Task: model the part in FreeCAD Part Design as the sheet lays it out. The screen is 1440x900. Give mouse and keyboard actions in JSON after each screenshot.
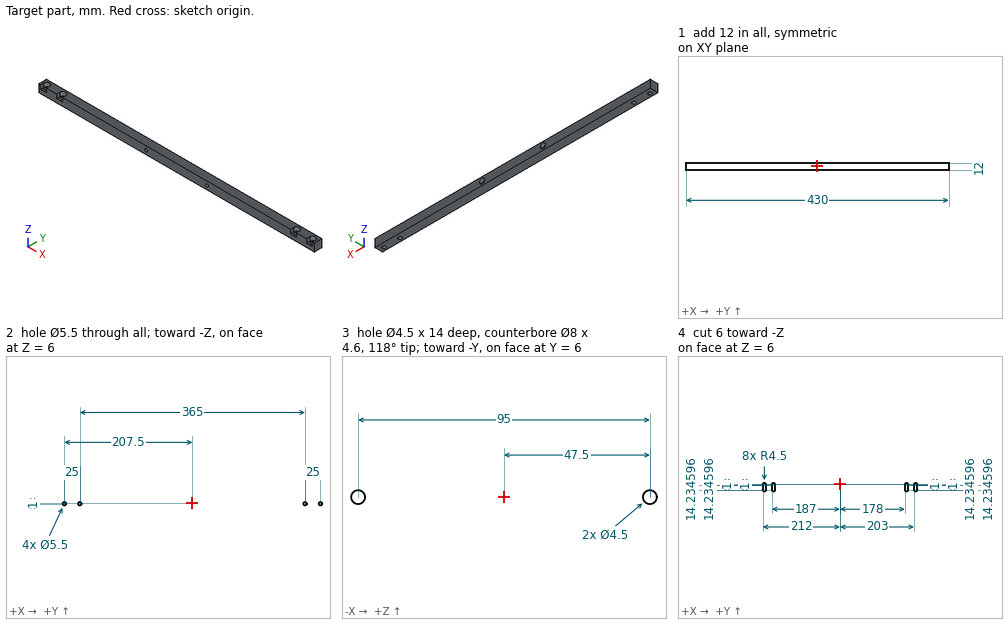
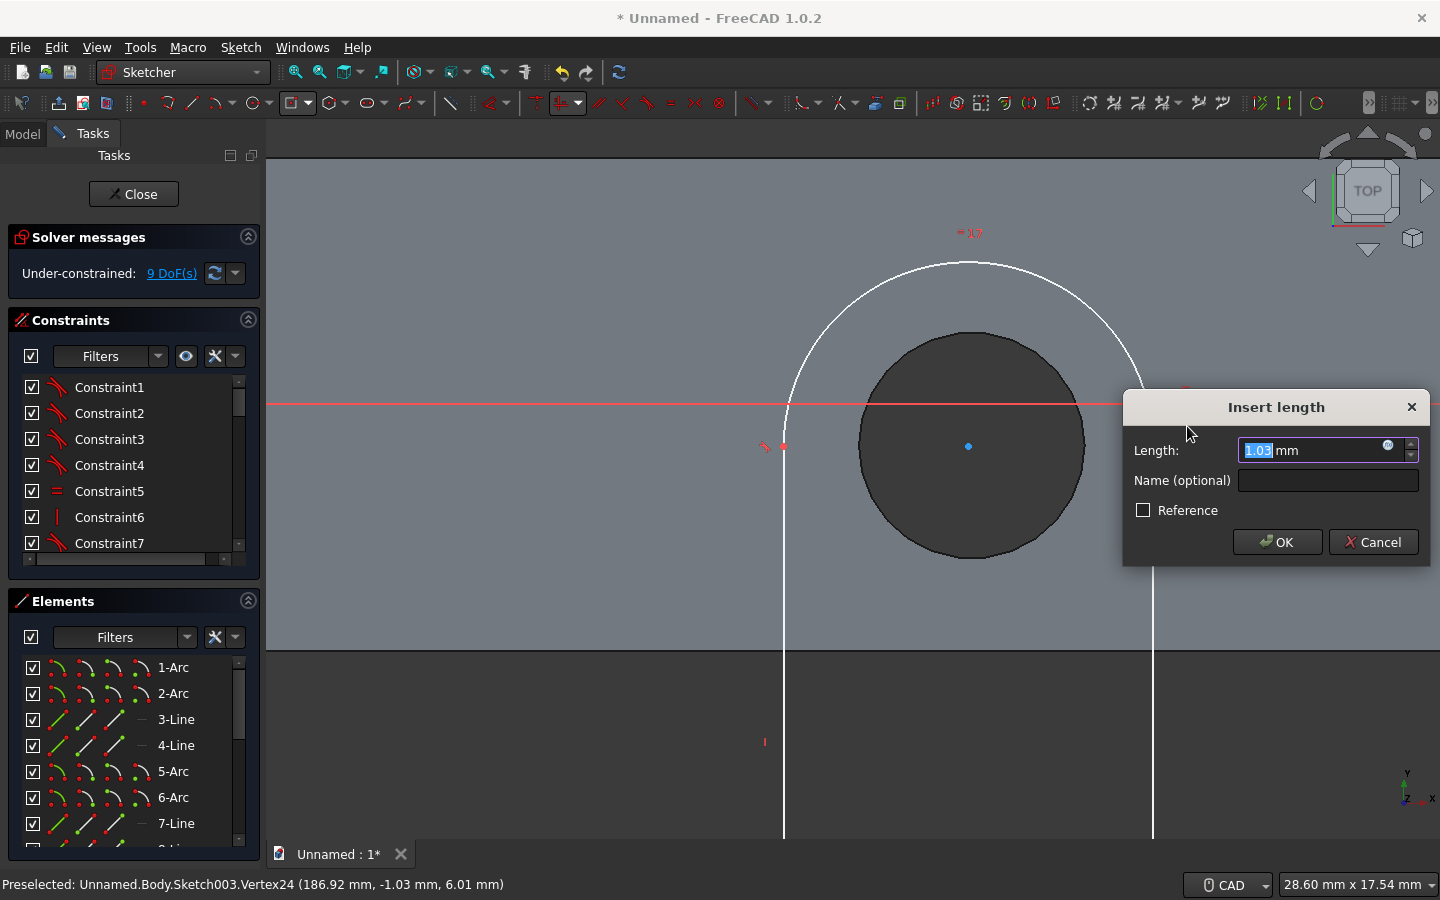
{"action": "type", "text": "1"}
{"action": "key", "text": "Return"}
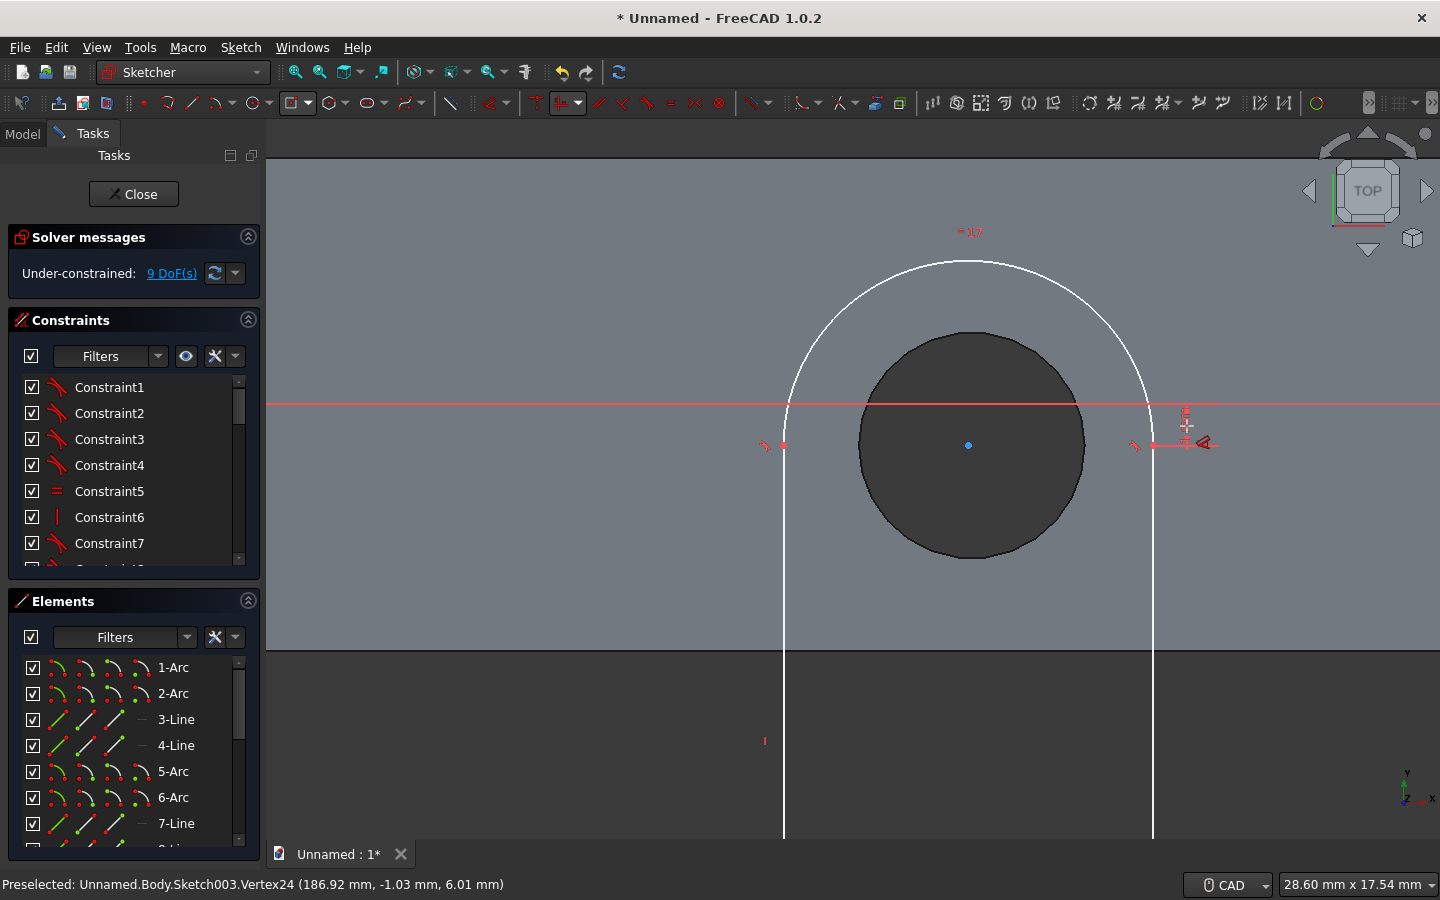
{"action": "scroll", "coordinate": [1167, 465], "scroll_direction": "down", "scroll_amount": 15}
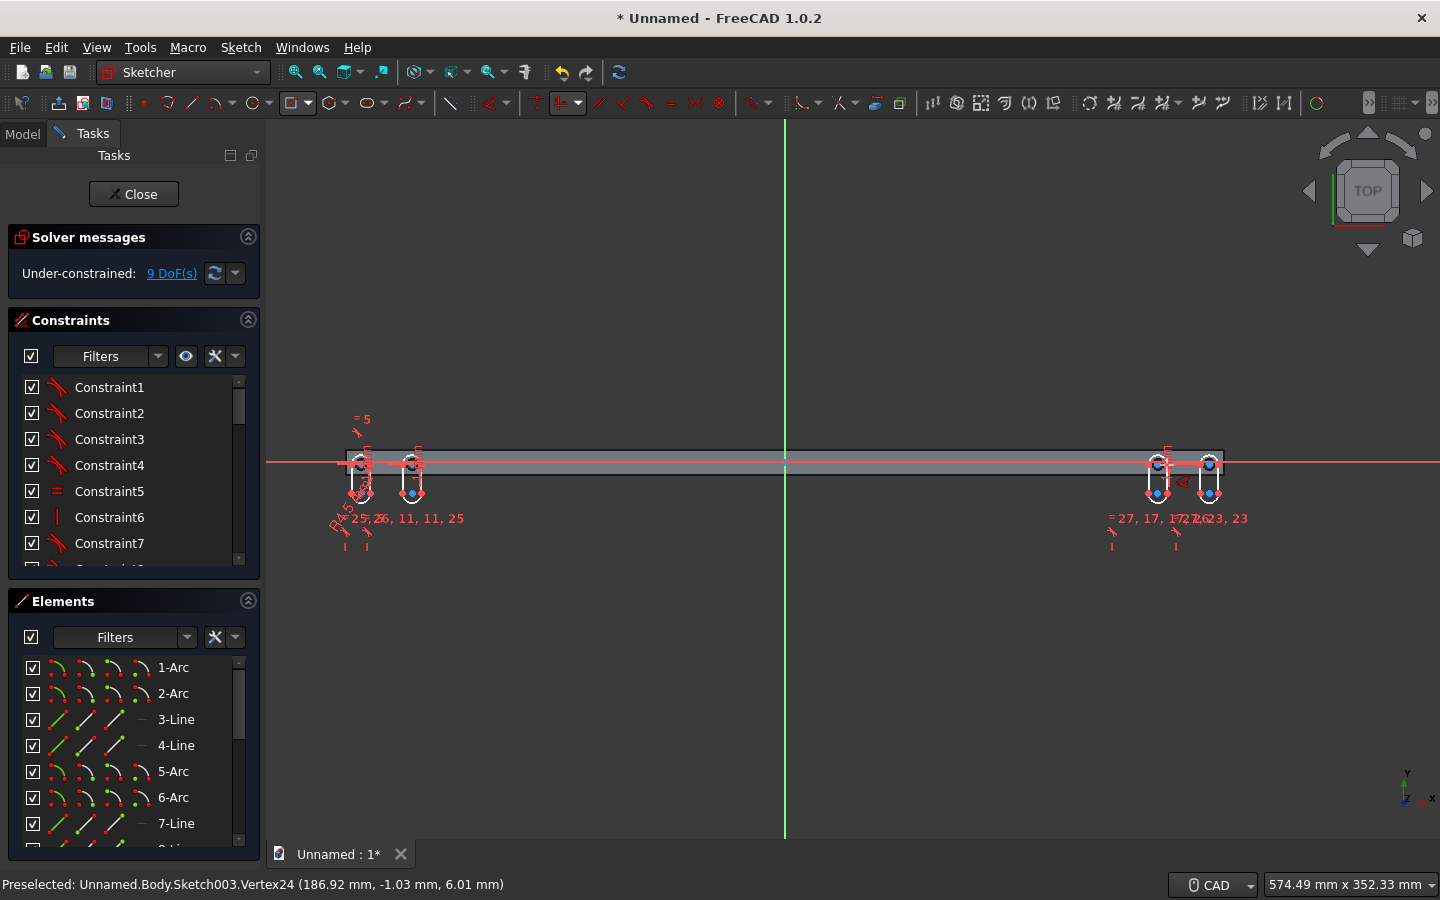
{"action": "scroll", "coordinate": [1218, 465], "scroll_direction": "up", "scroll_amount": 15}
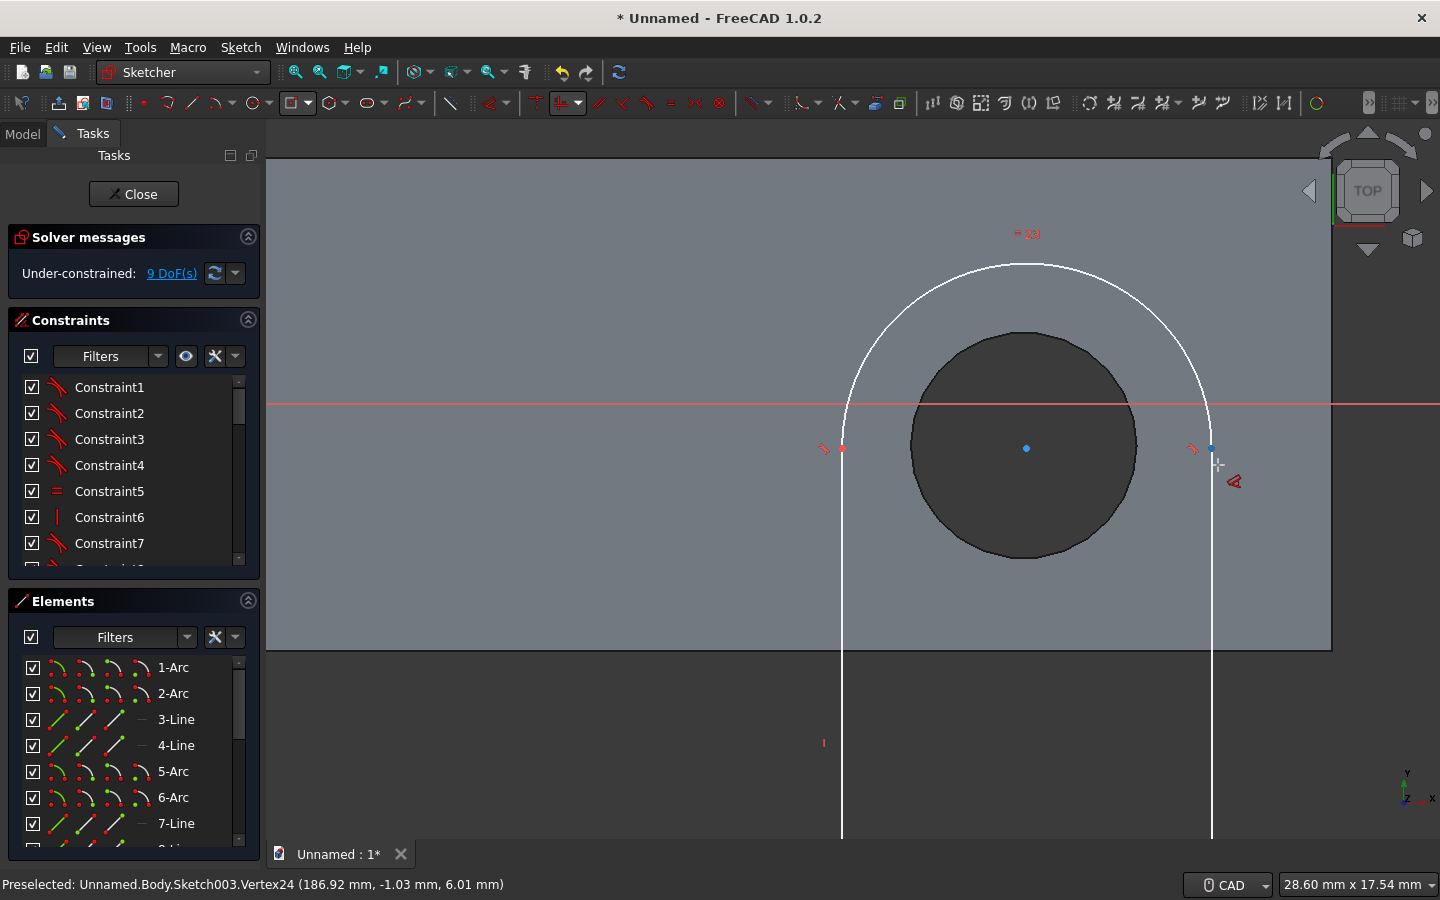
{"action": "left_click", "coordinate": [1212, 448]}
{"action": "left_click", "coordinate": [1246, 426]}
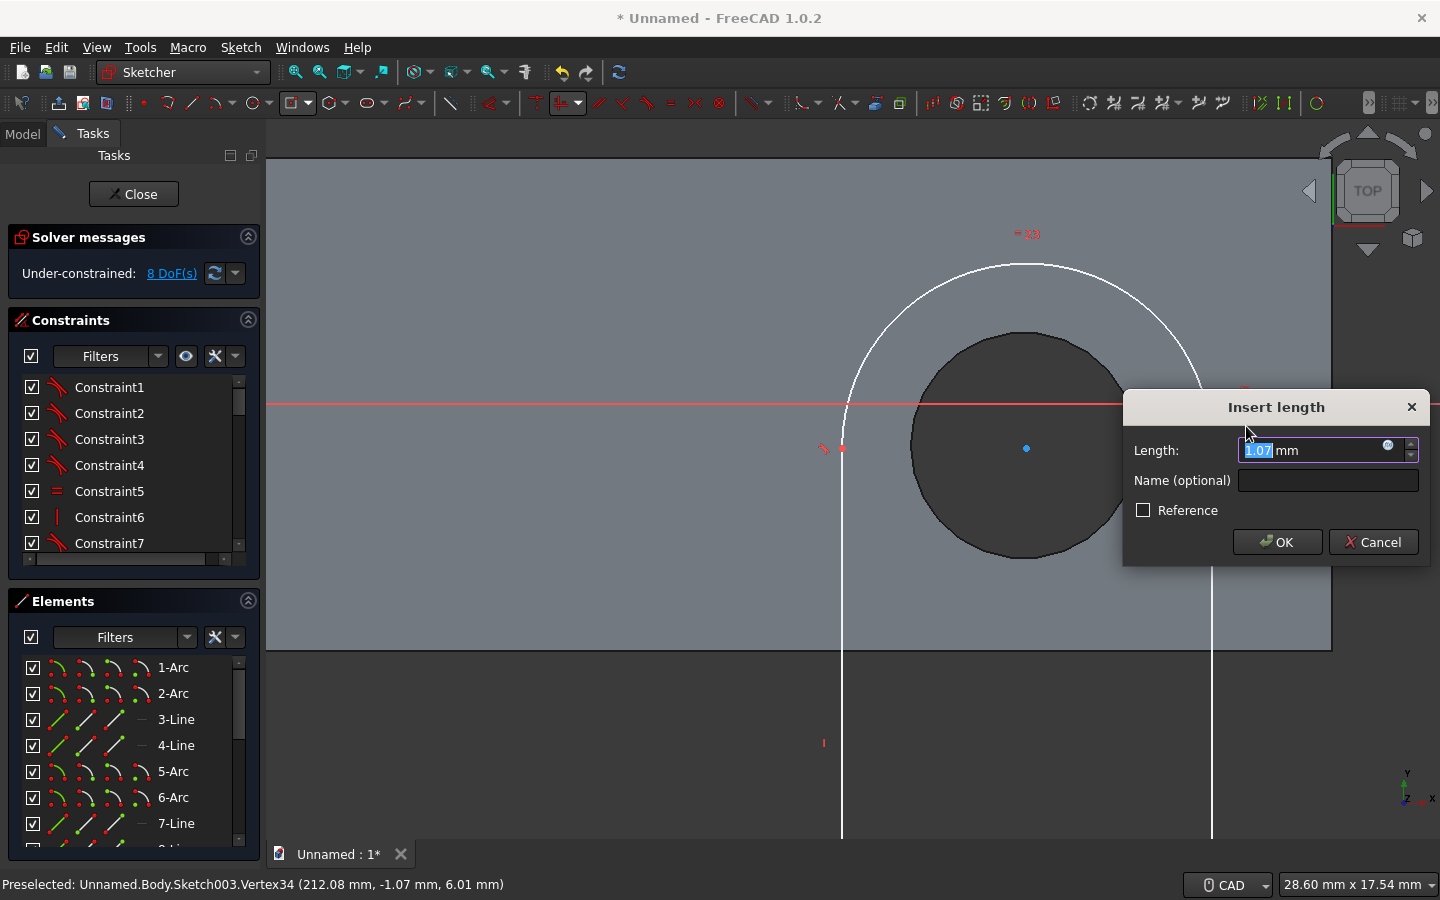
{"action": "type", "text": "1"}
{"action": "key", "text": "Return"}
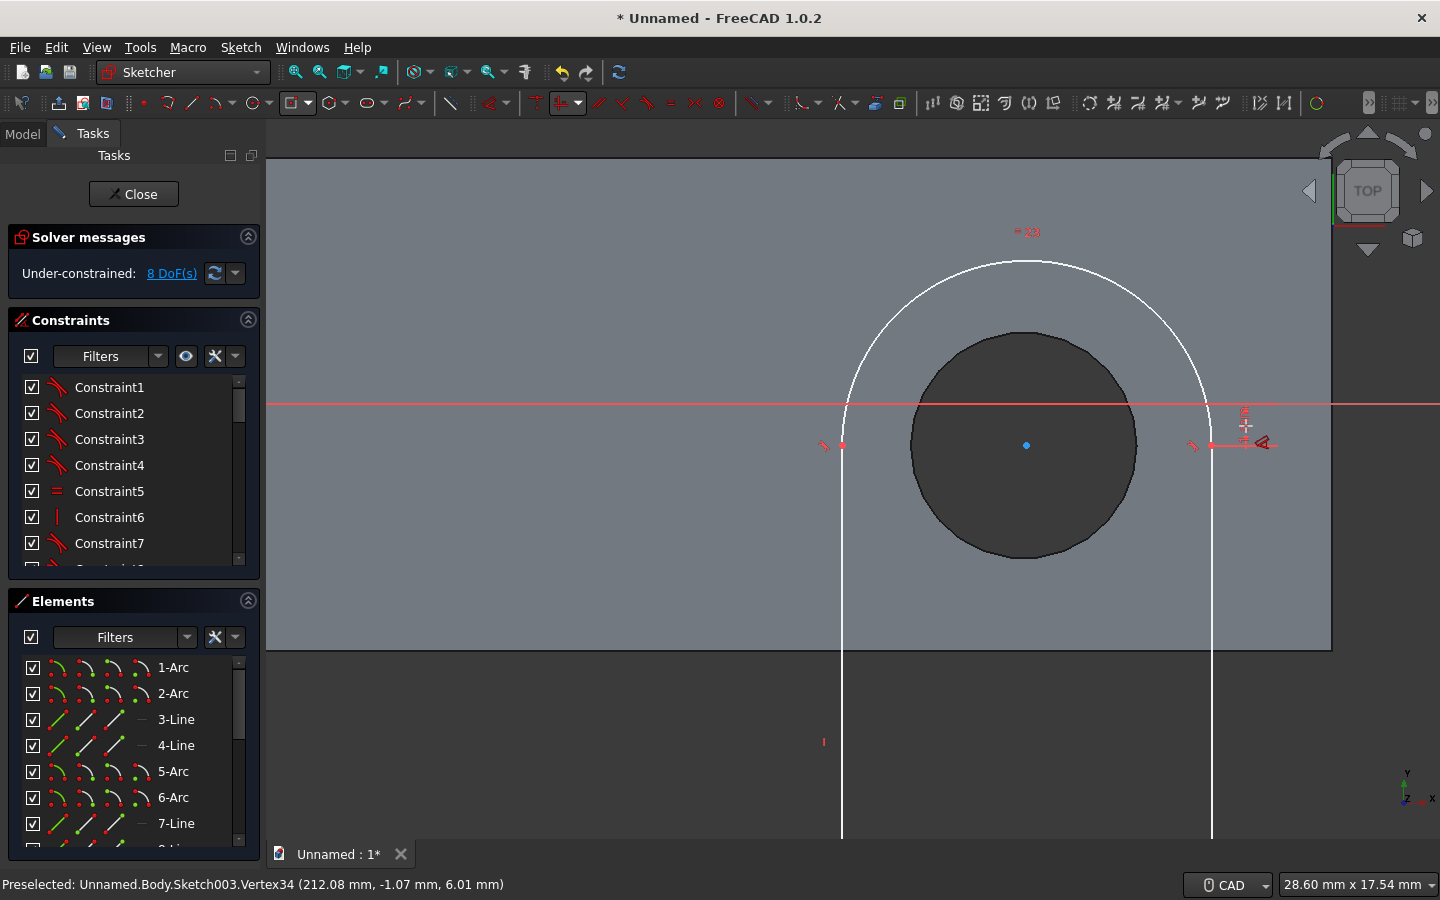
{"action": "scroll", "coordinate": [1218, 465], "scroll_direction": "down", "scroll_amount": 15}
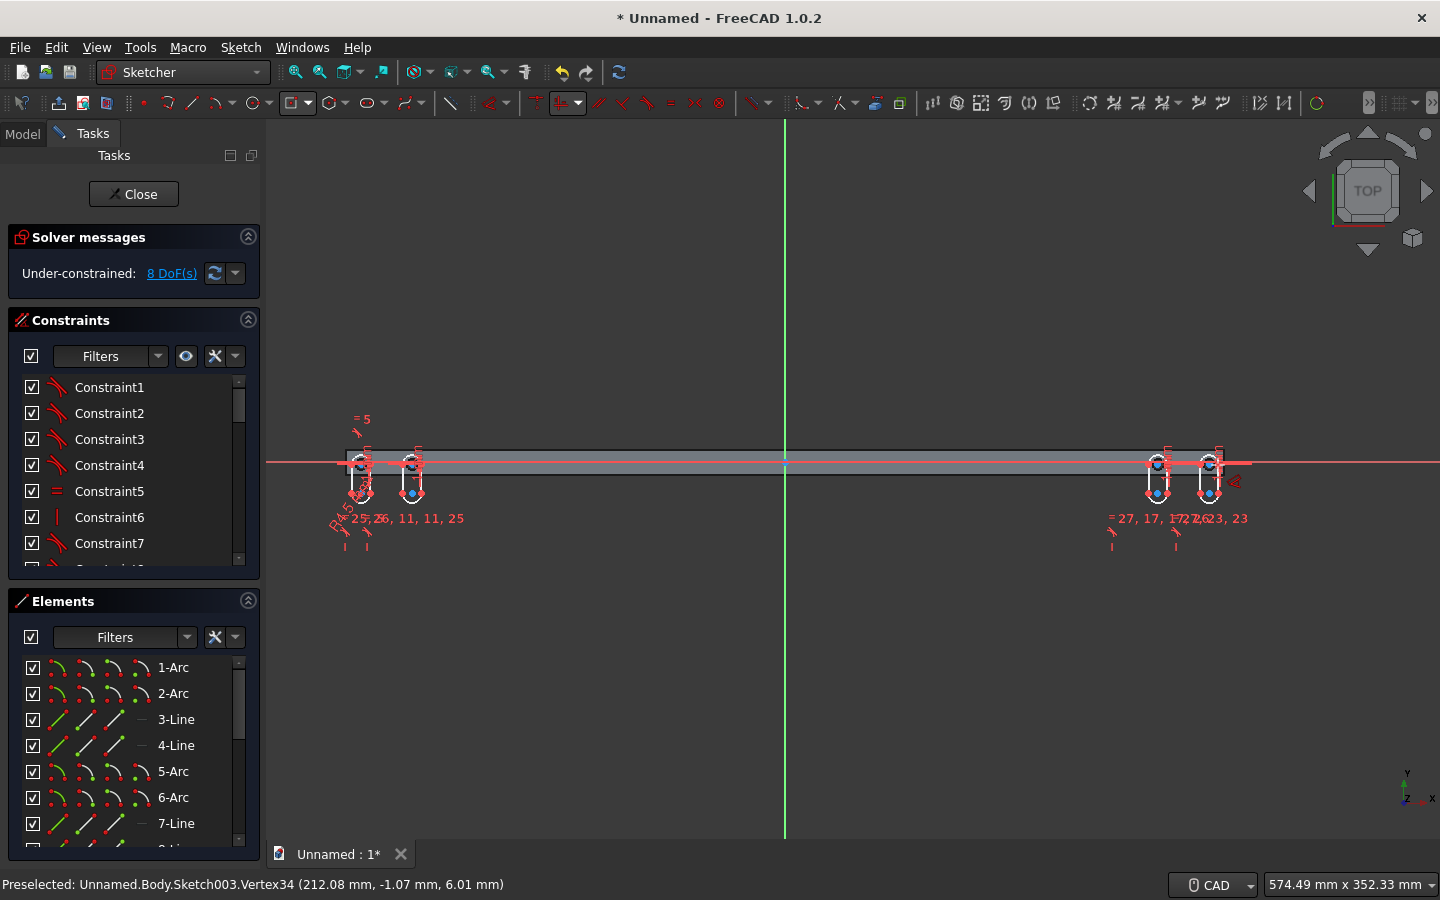
{"action": "scroll", "coordinate": [352, 494], "scroll_direction": "up", "scroll_amount": 2}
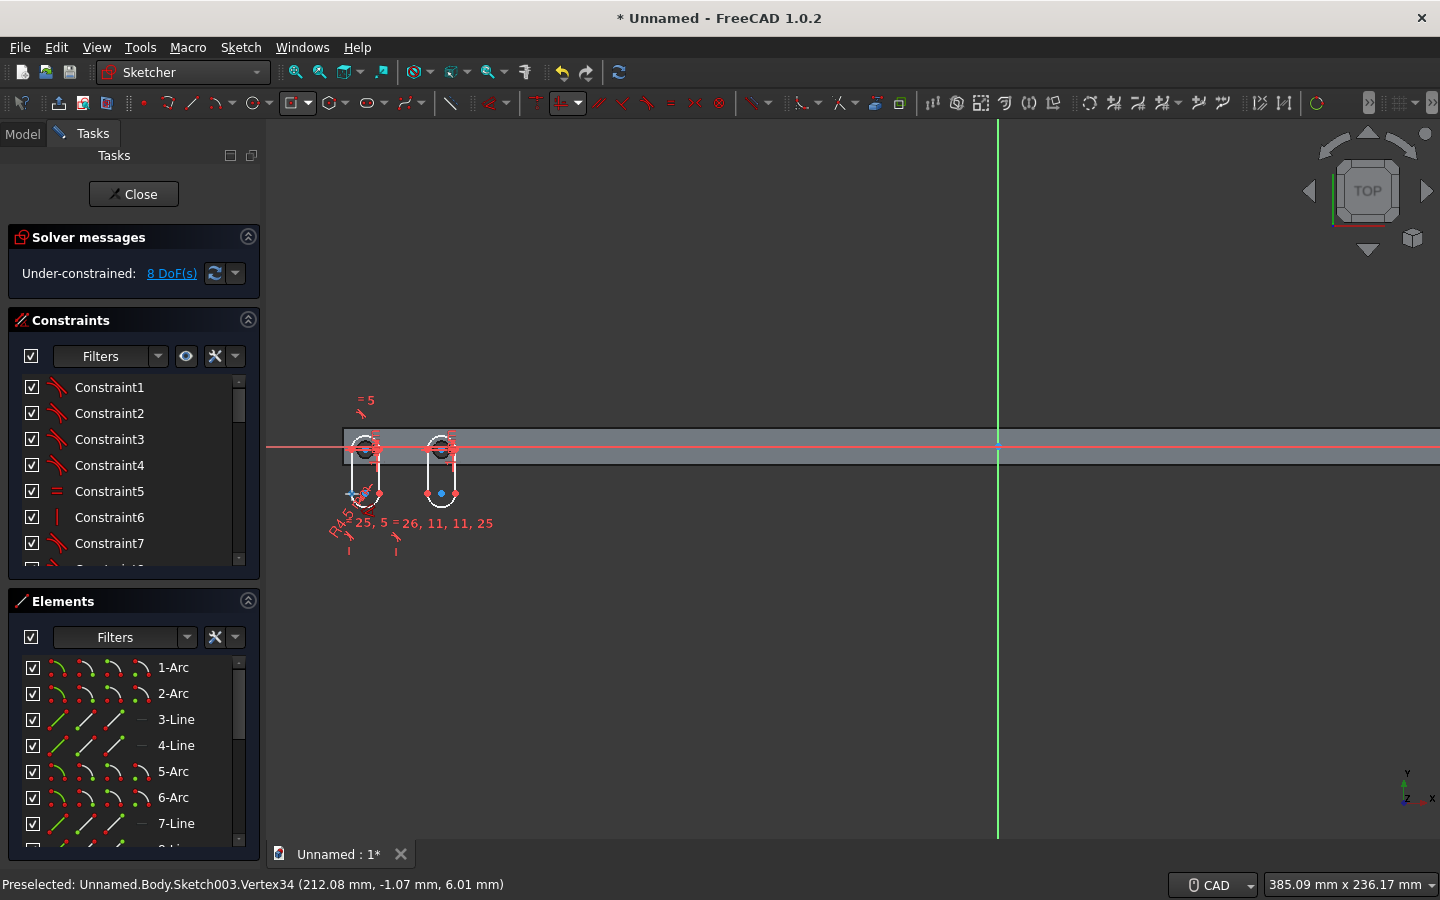
{"action": "left_click", "coordinate": [352, 493]}
{"action": "left_click", "coordinate": [675, 413]}